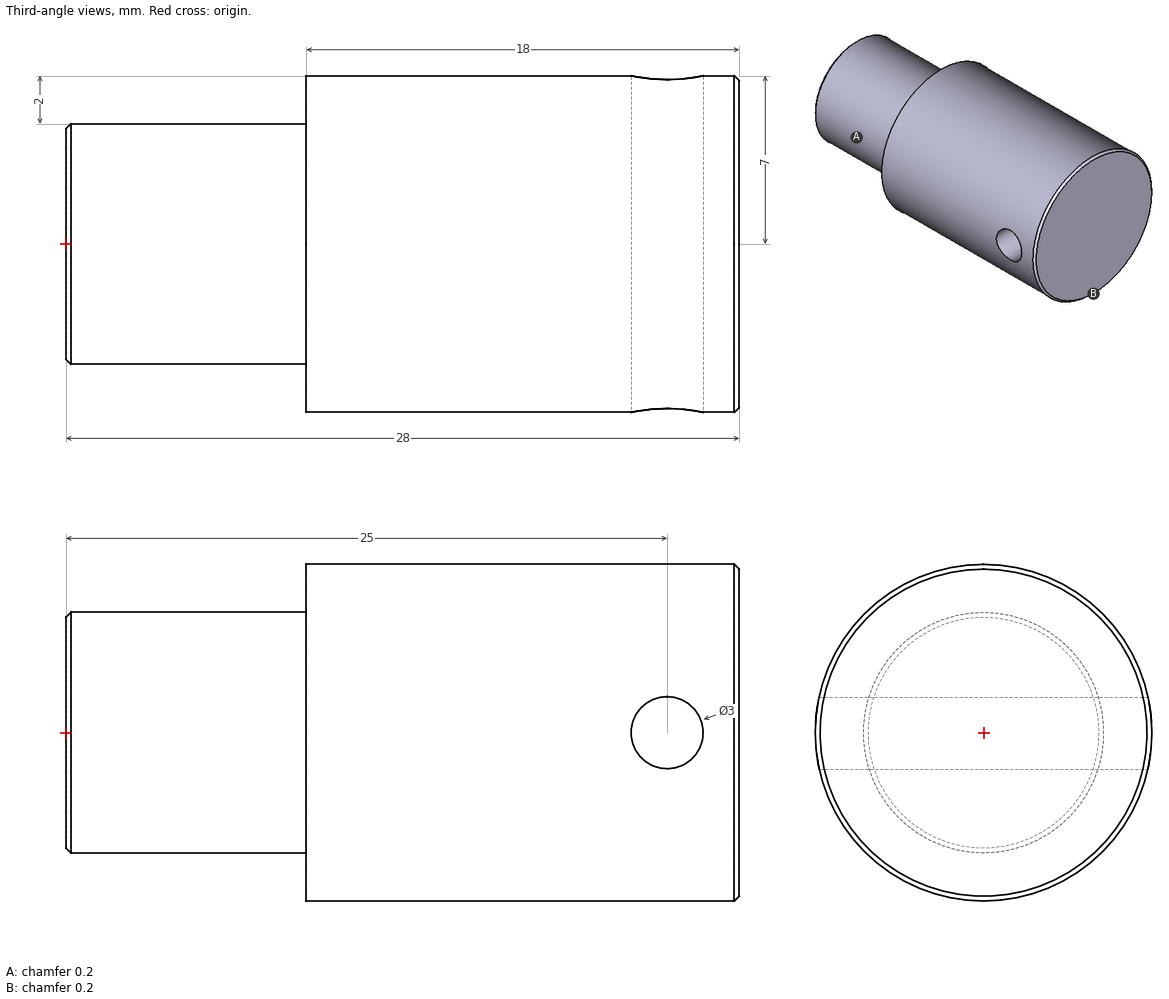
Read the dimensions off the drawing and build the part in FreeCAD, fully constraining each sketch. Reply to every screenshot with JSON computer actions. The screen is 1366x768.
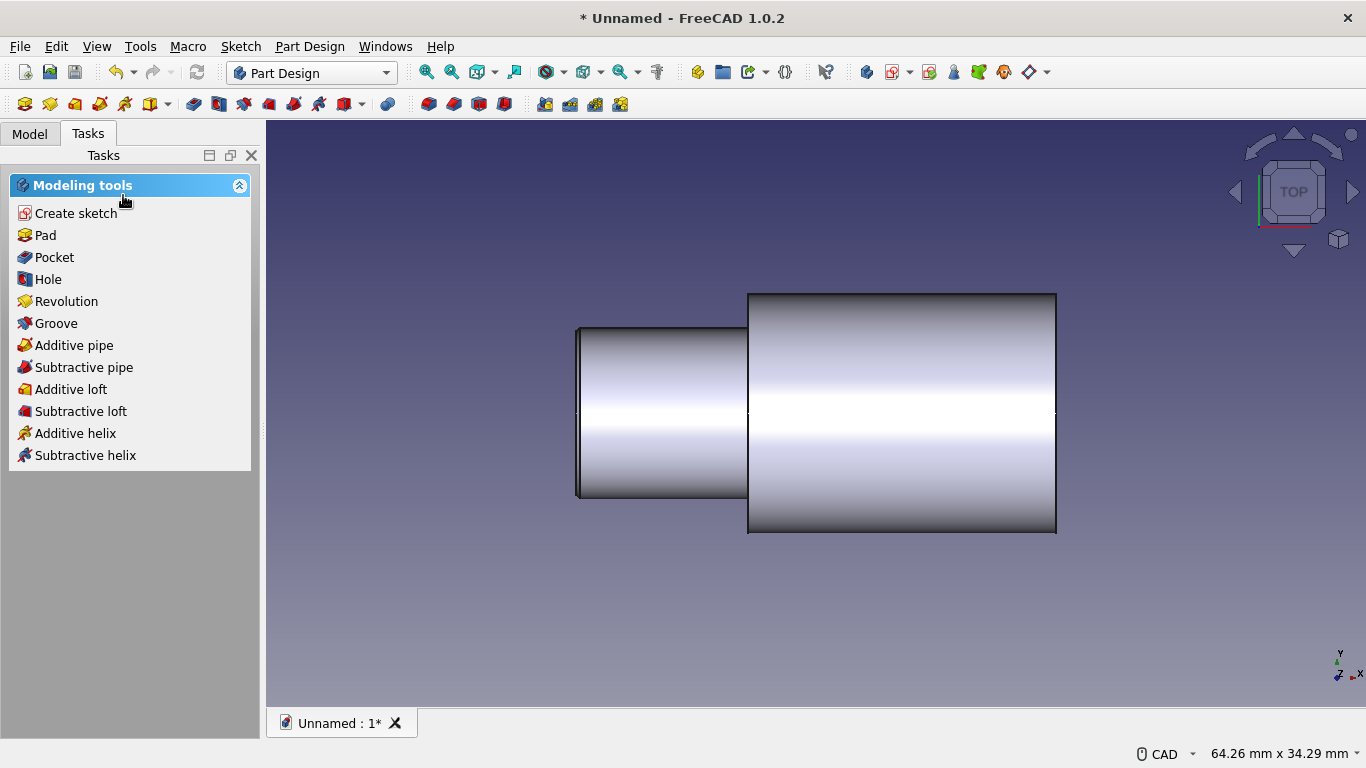
{"action": "left_click", "coordinate": [194, 104]}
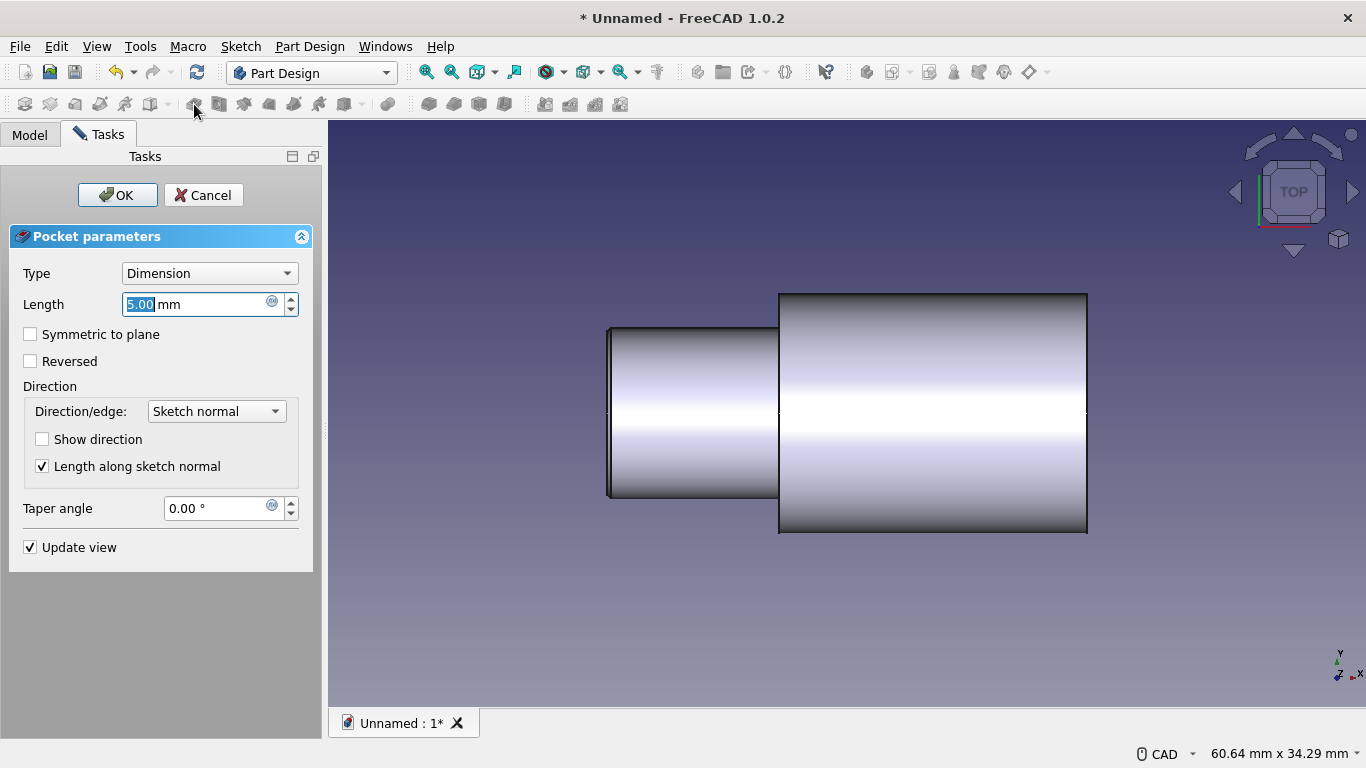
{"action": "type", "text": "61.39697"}
{"action": "key", "text": "Tab"}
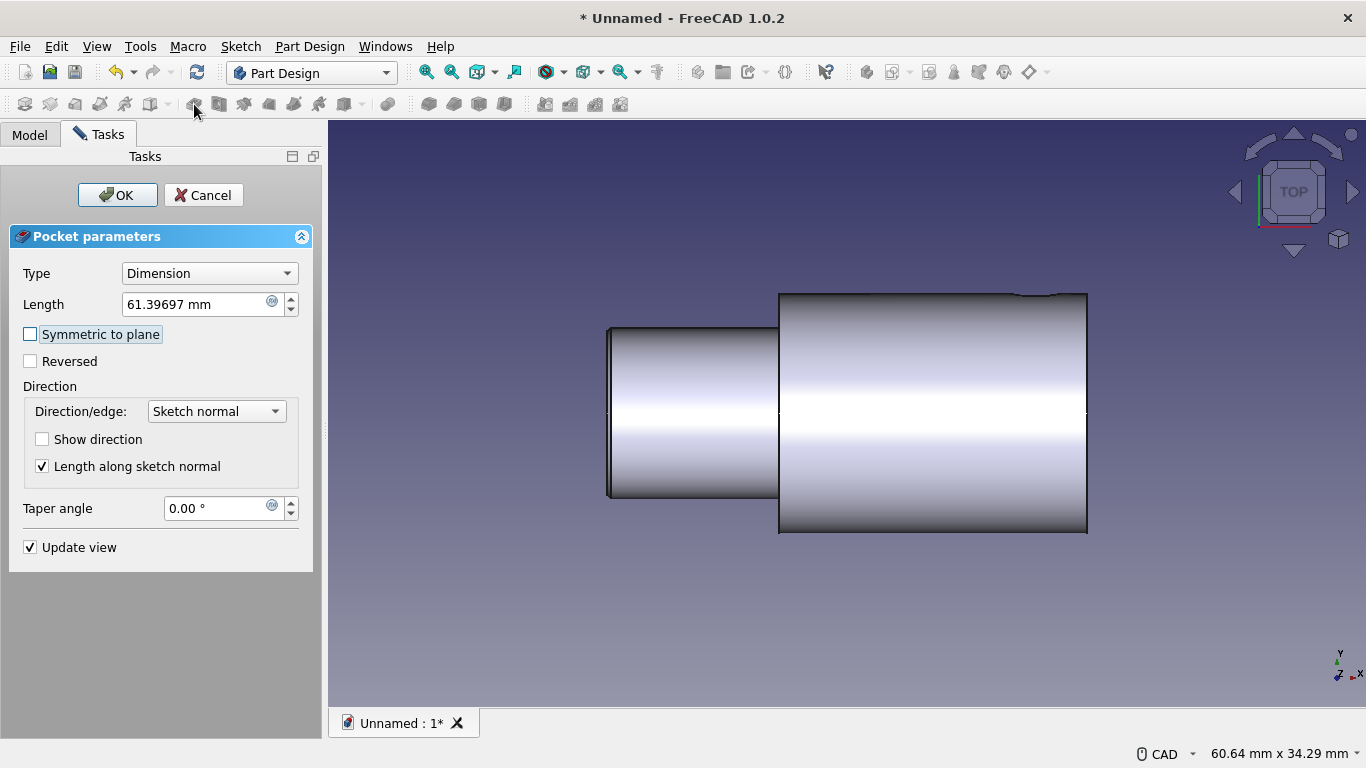
{"action": "left_click", "coordinate": [31, 334]}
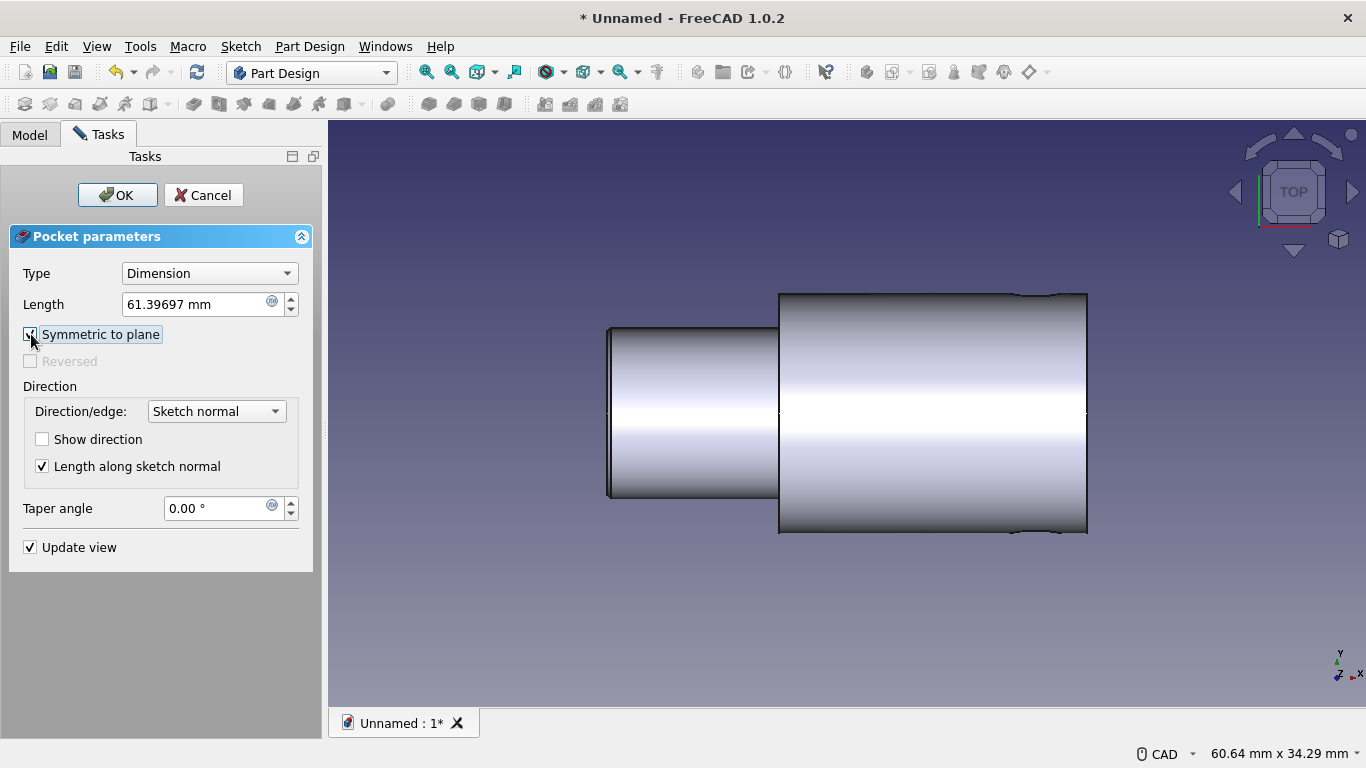
{"action": "left_click", "coordinate": [118, 195]}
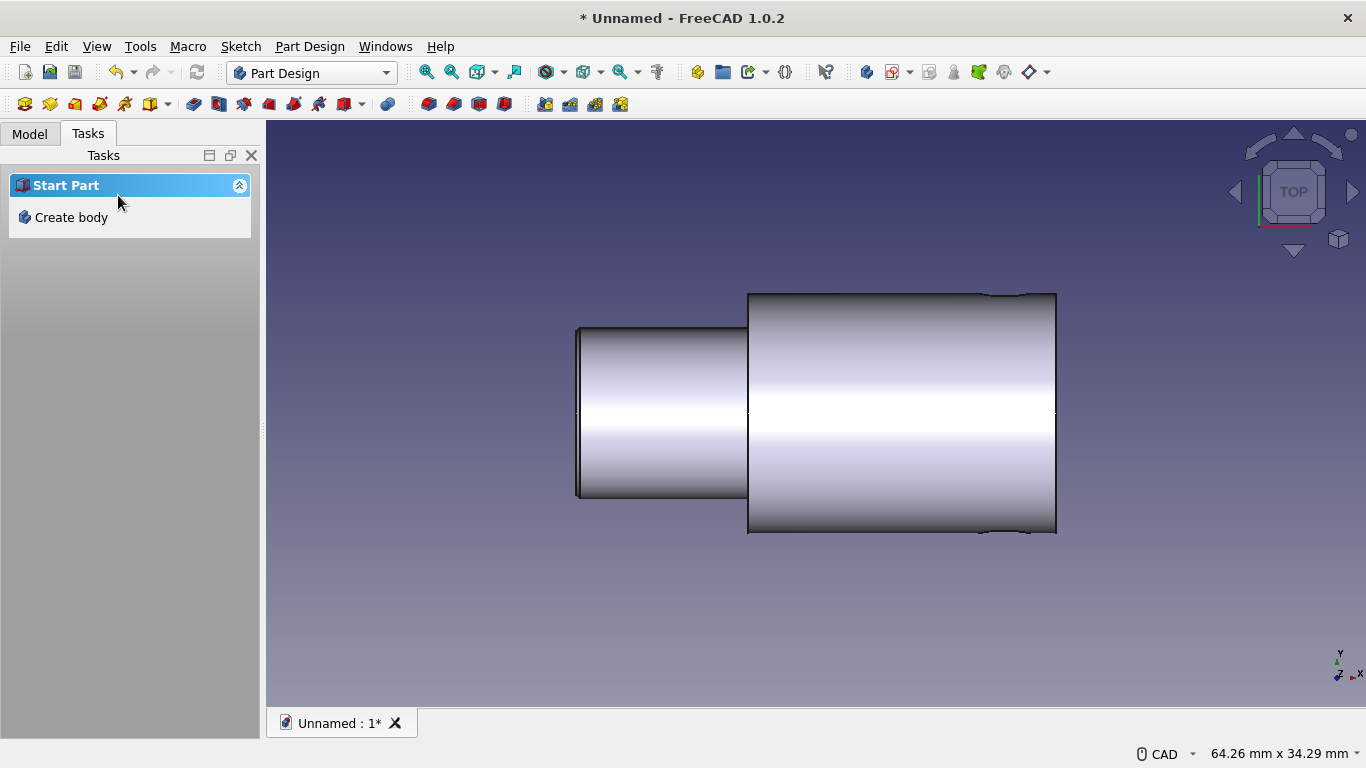
{"action": "left_click", "coordinate": [427, 72]}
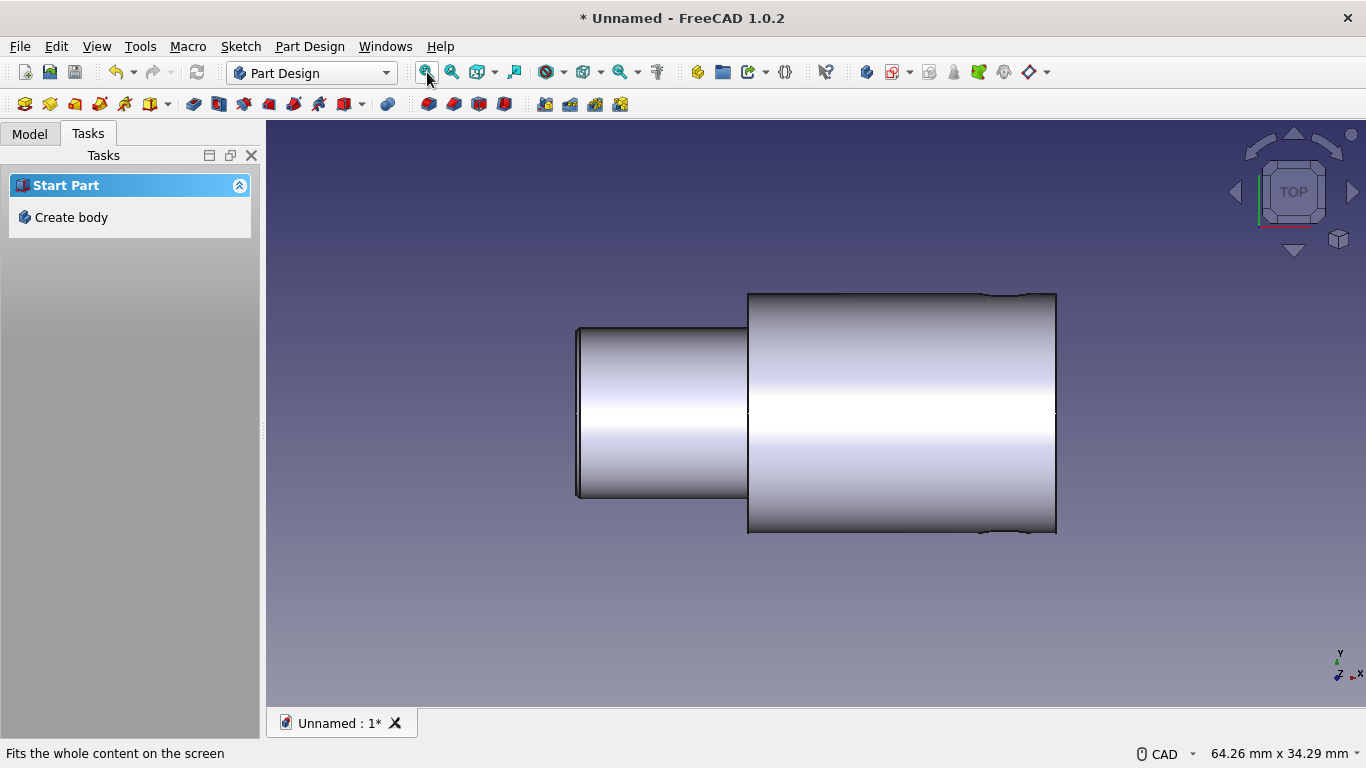
{"action": "left_click", "coordinate": [1056, 509]}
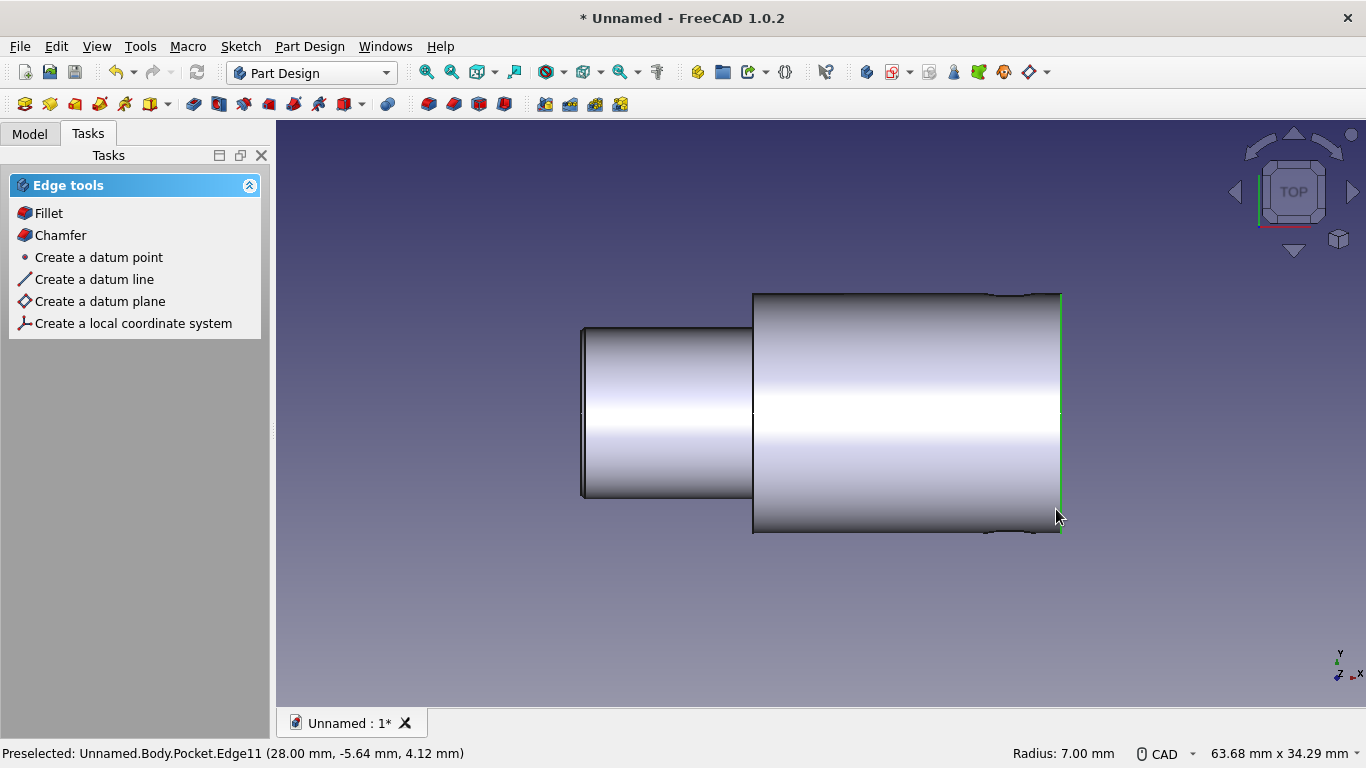
{"action": "left_click", "coordinate": [454, 104]}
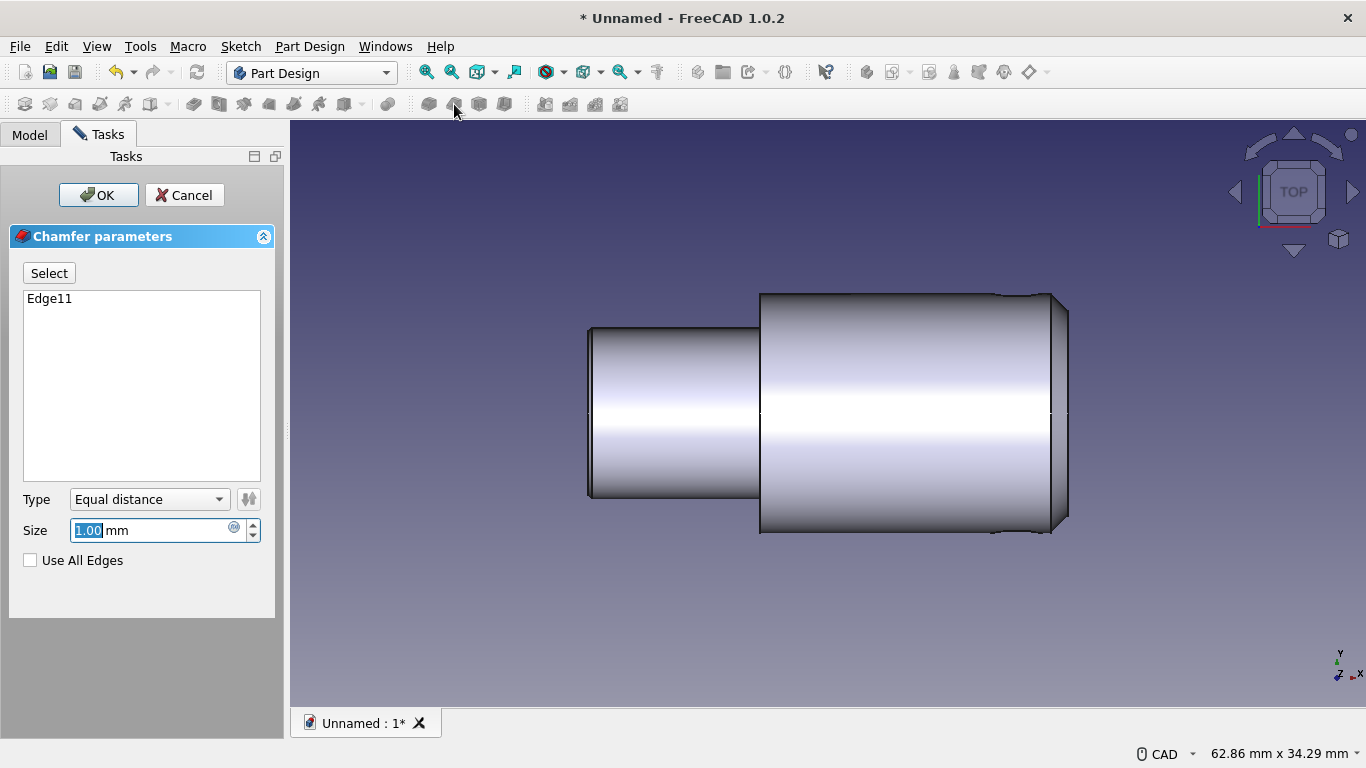
{"action": "type", "text": "0.2"}
{"action": "key", "text": "Tab"}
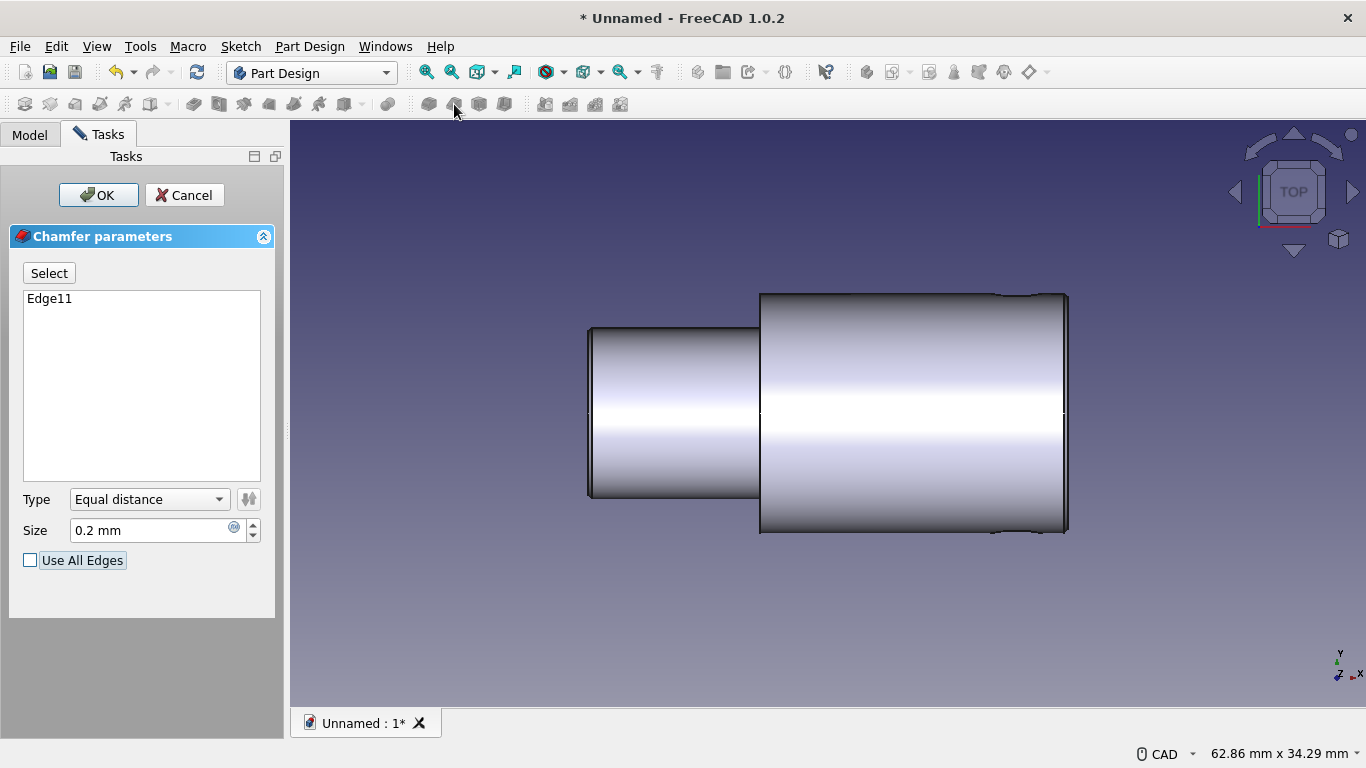
{"action": "left_click", "coordinate": [99, 195]}